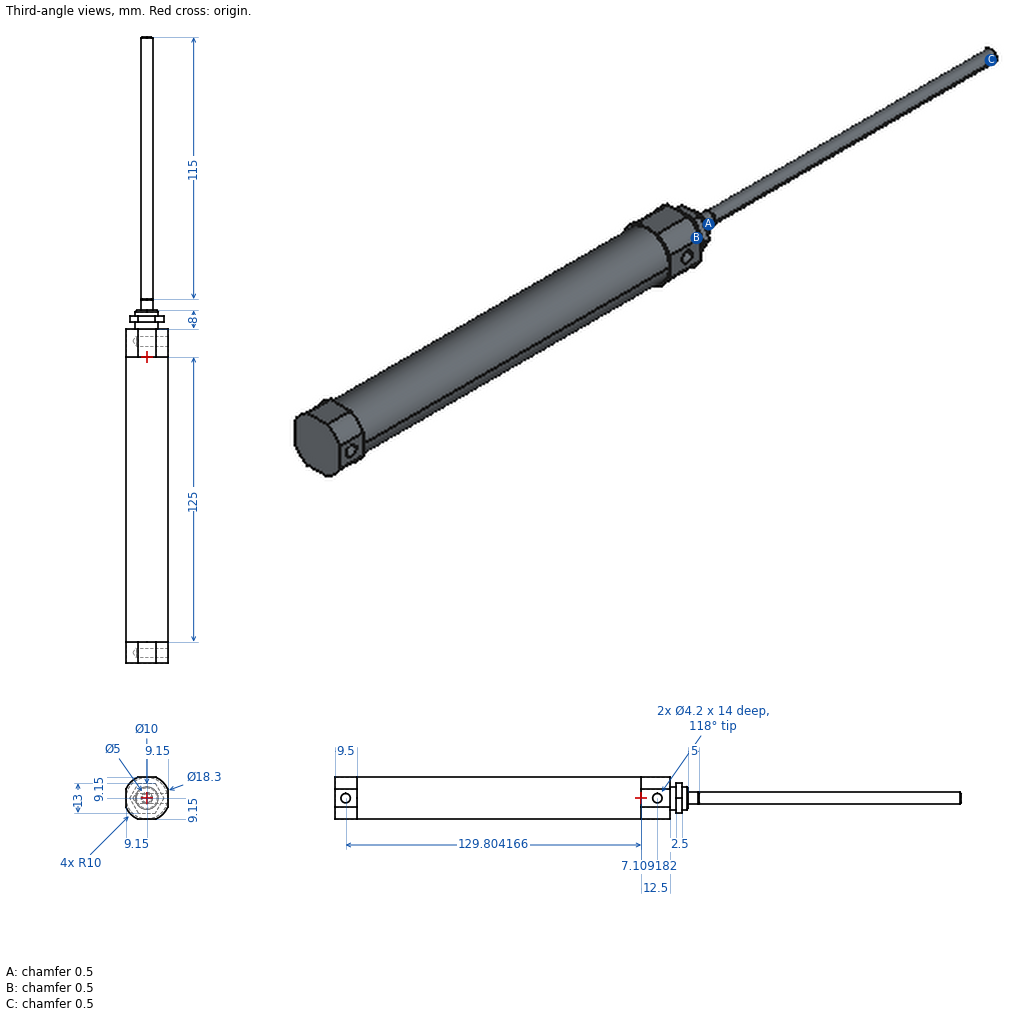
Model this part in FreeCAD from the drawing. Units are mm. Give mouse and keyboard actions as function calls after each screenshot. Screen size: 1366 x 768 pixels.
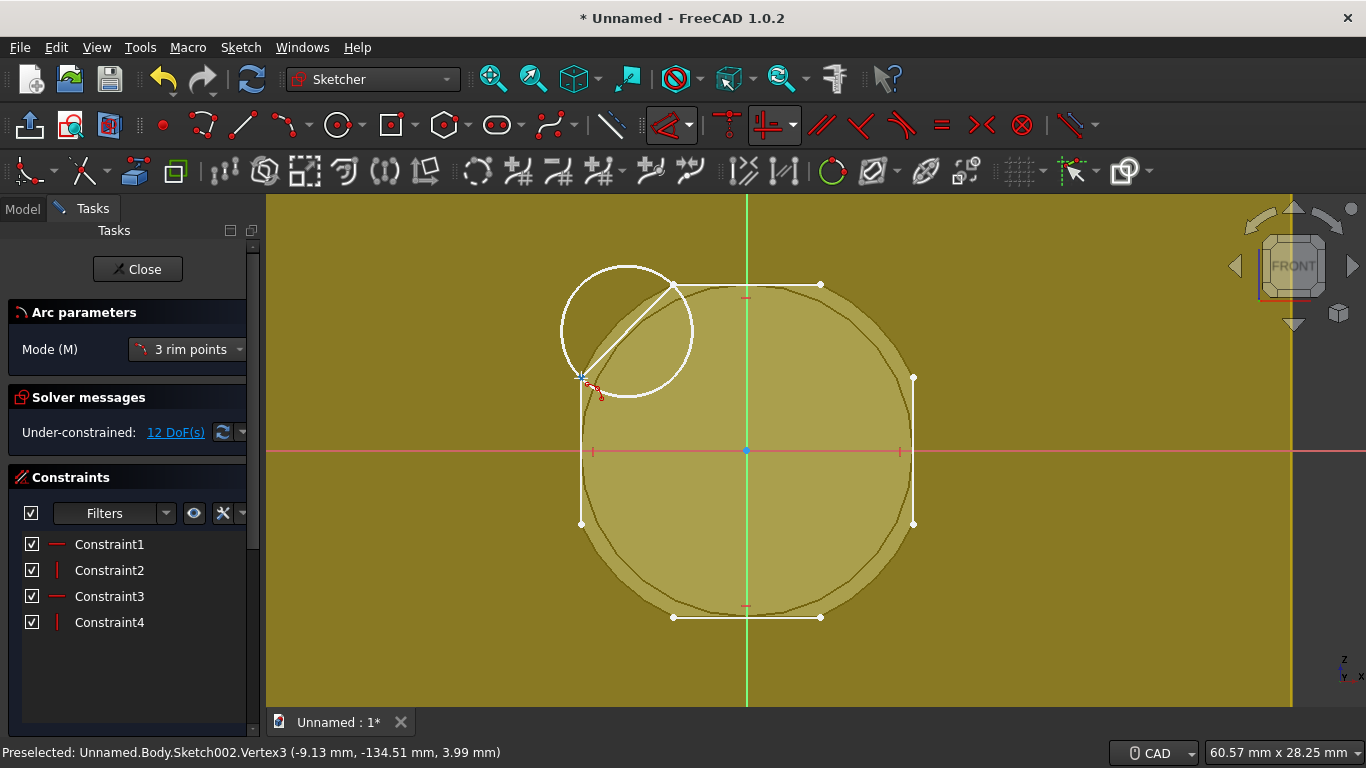
scroll(618, 322, up, 2)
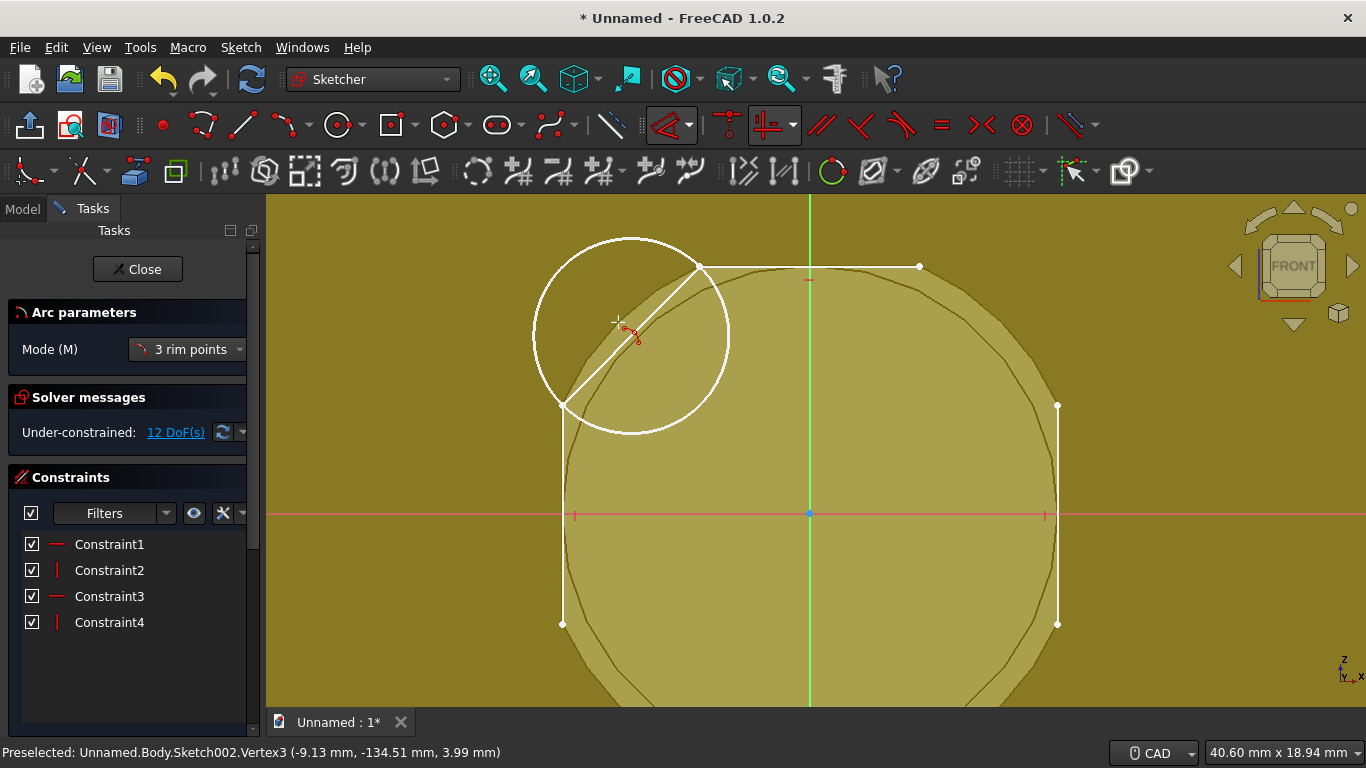
click(618, 322)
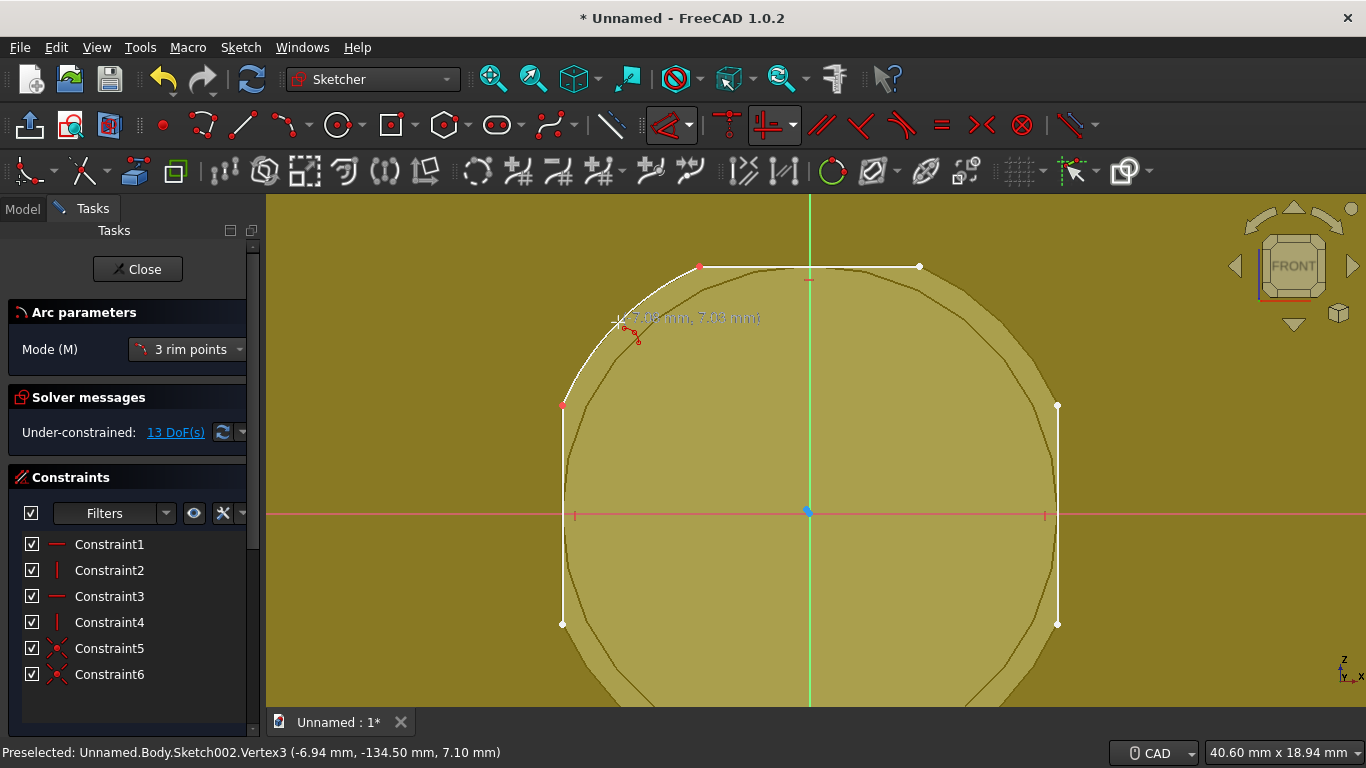
click(563, 625)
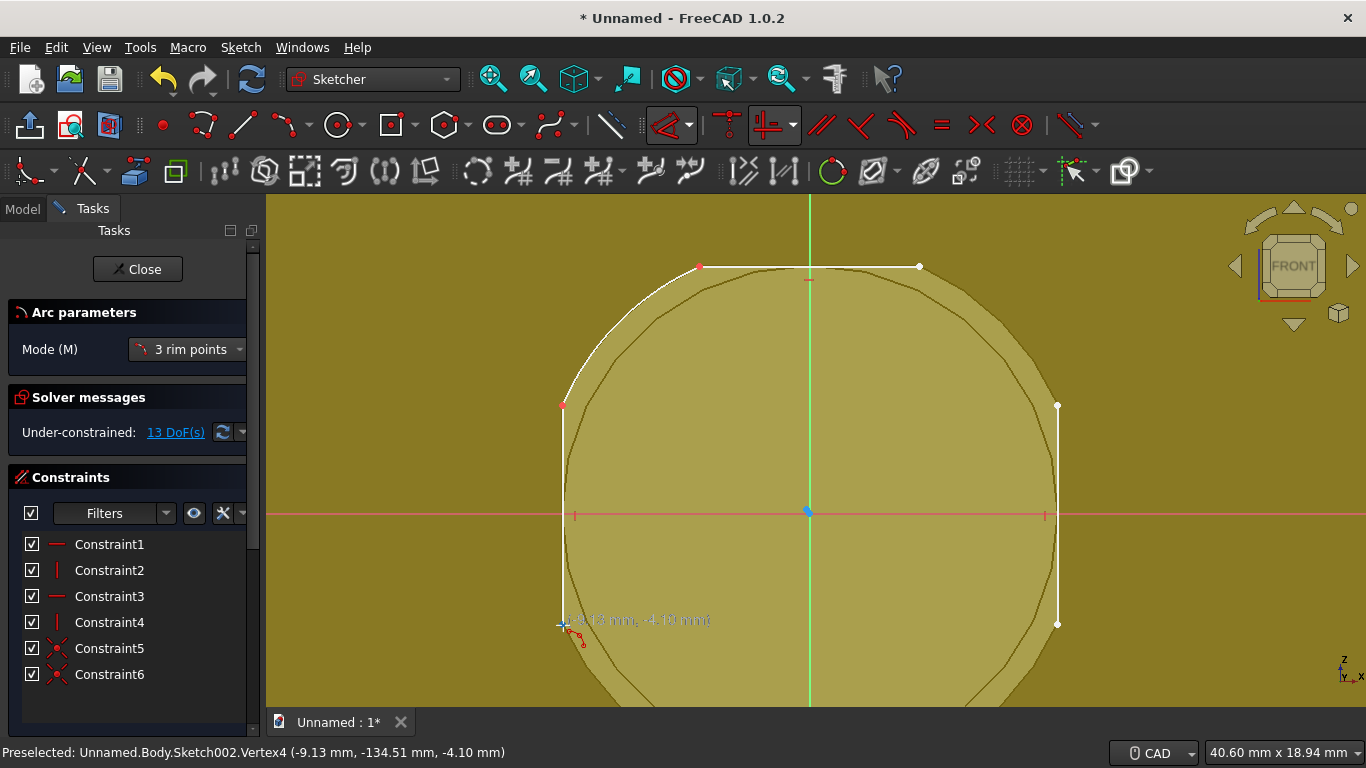
scroll(621, 322, down, 2)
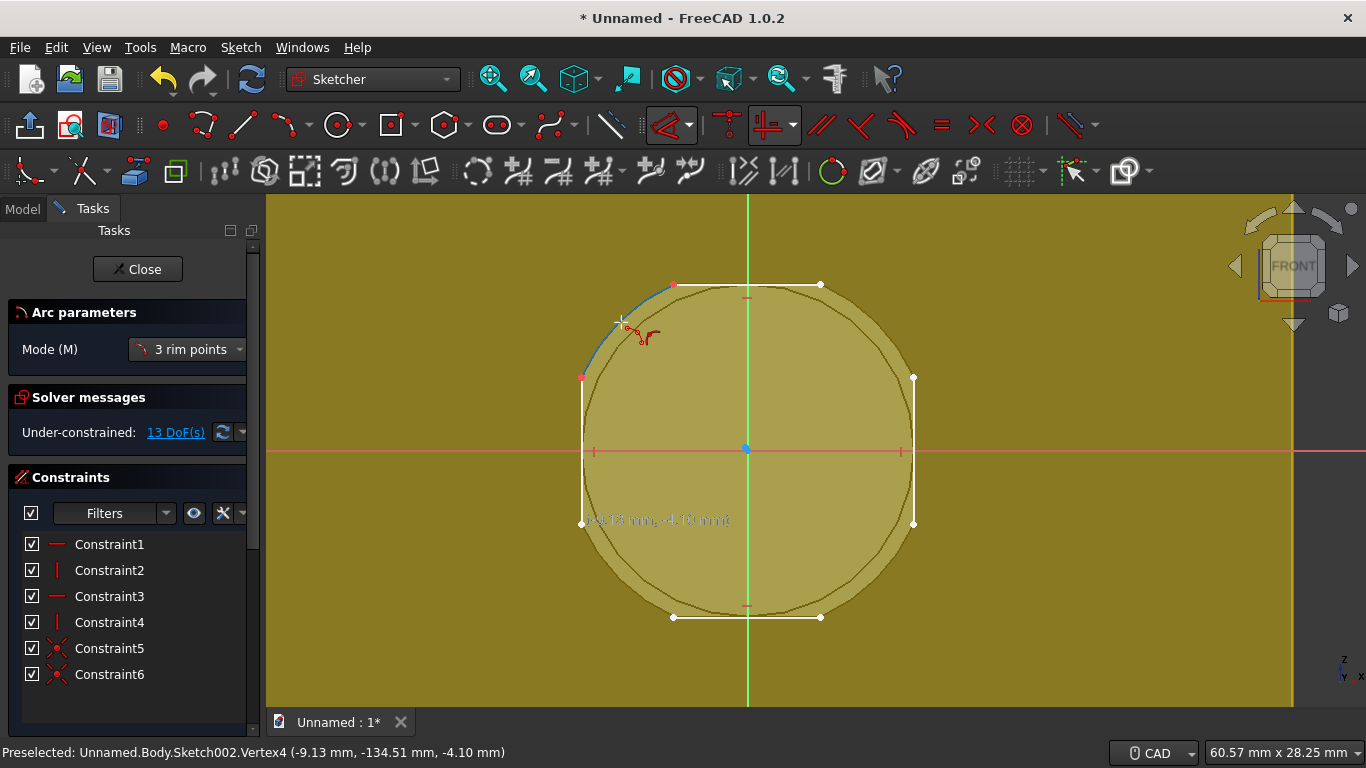
click(674, 618)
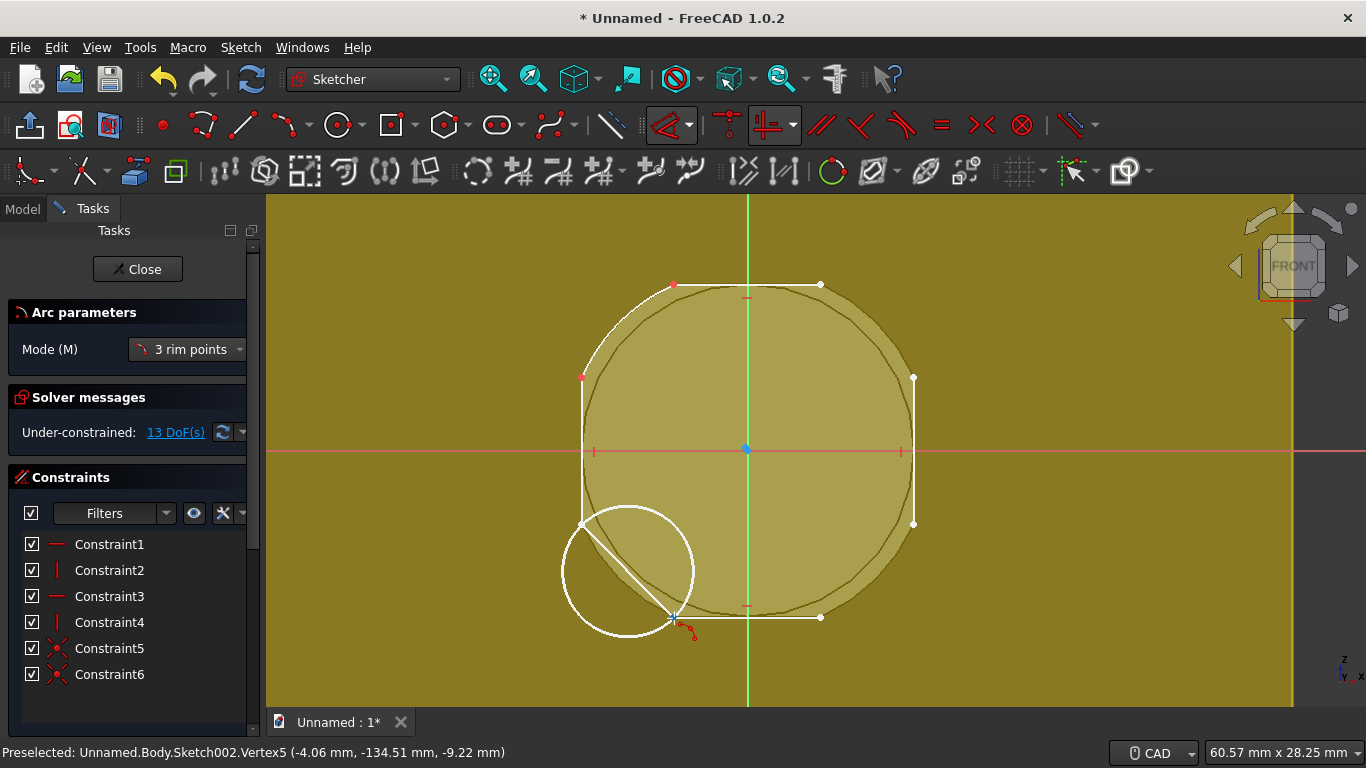
scroll(619, 579, up, 2)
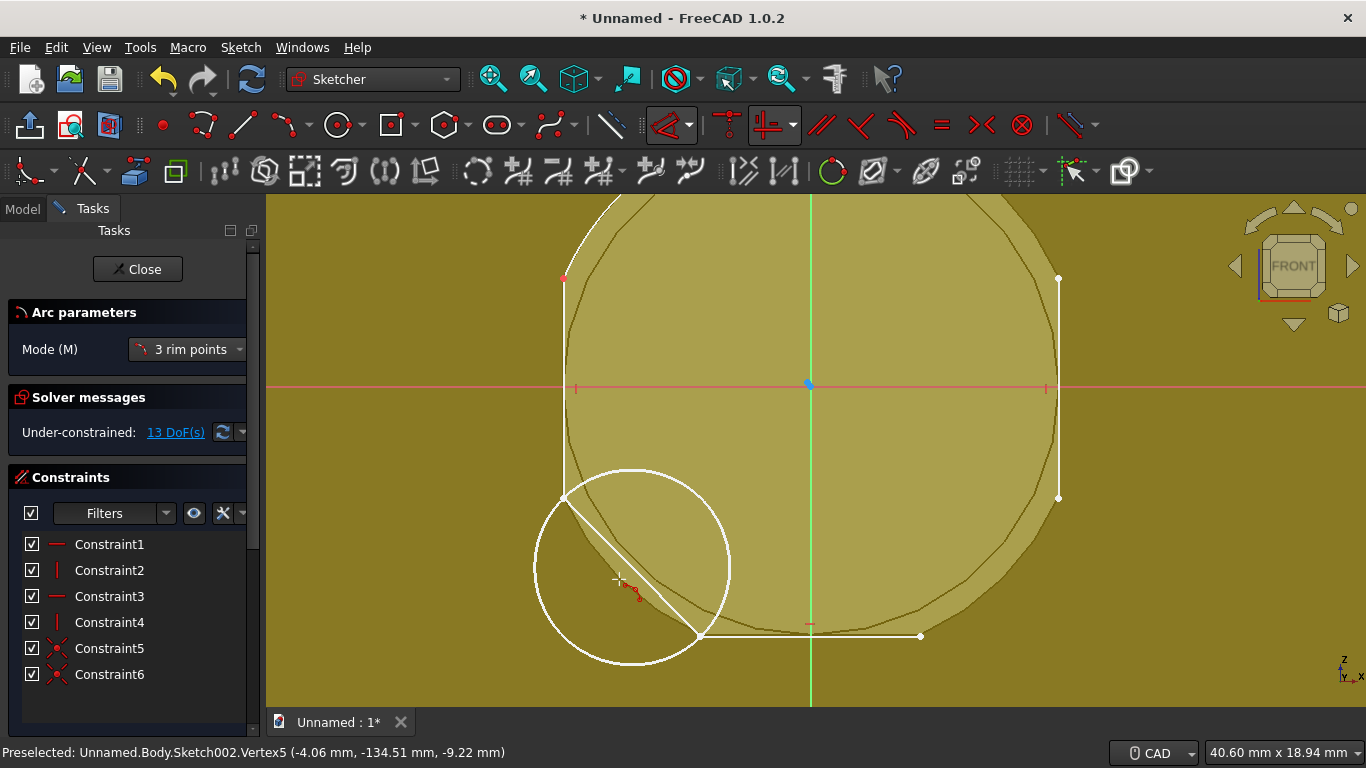
click(619, 579)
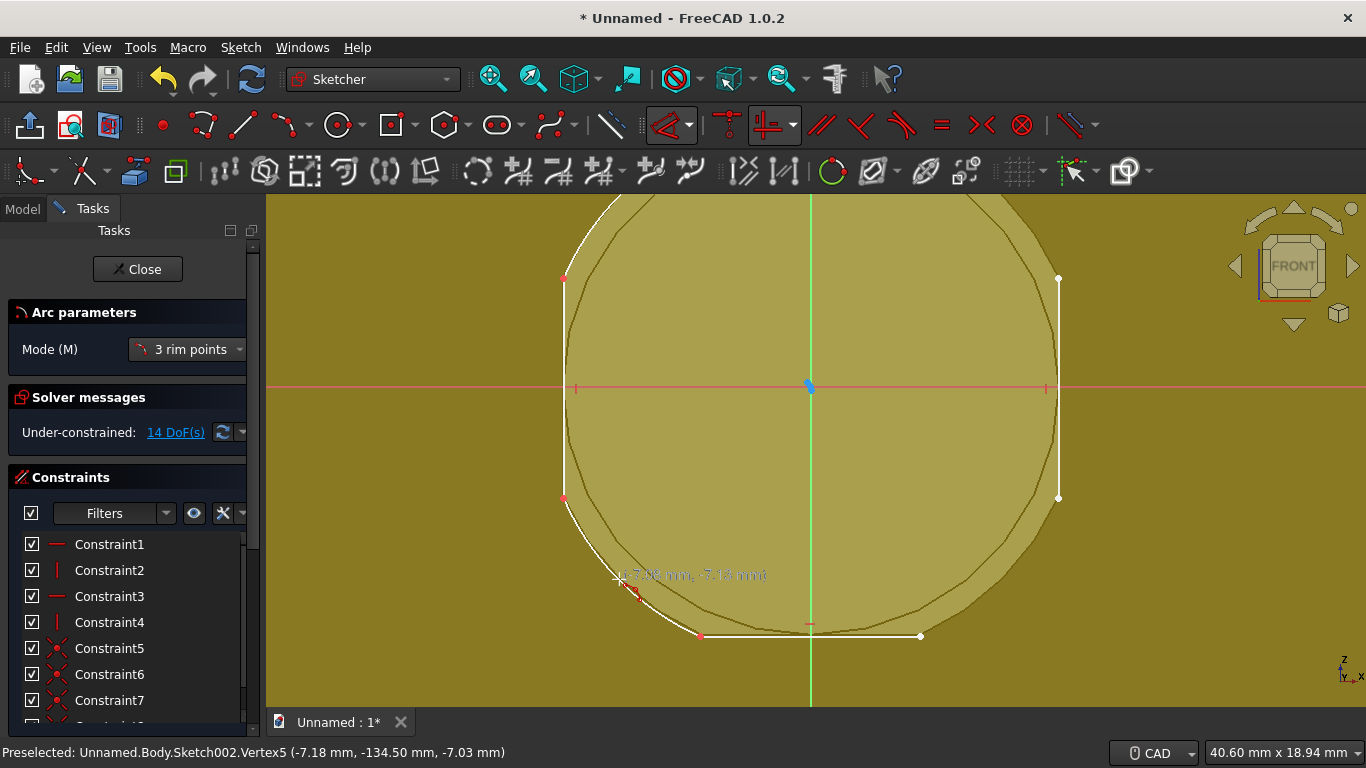
click(920, 637)
click(1059, 498)
click(1002, 579)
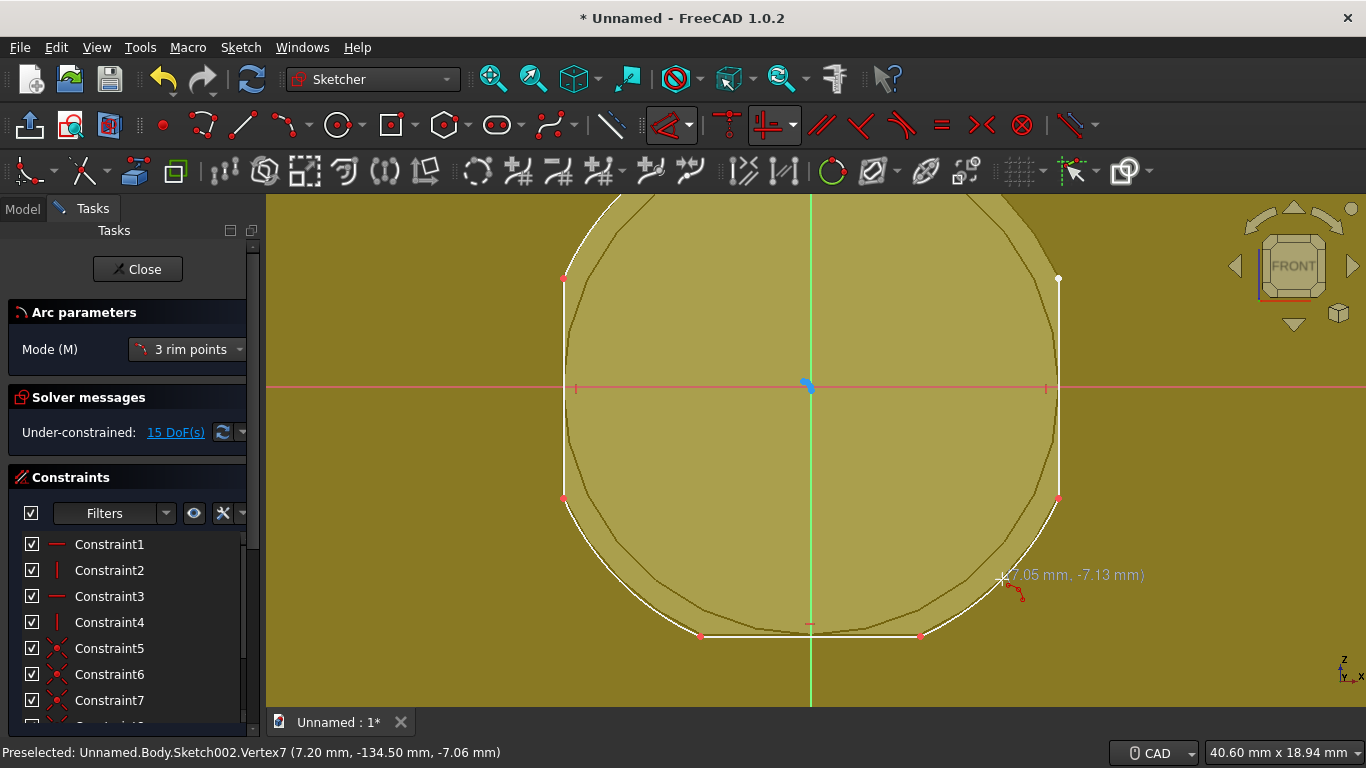
click(1059, 279)